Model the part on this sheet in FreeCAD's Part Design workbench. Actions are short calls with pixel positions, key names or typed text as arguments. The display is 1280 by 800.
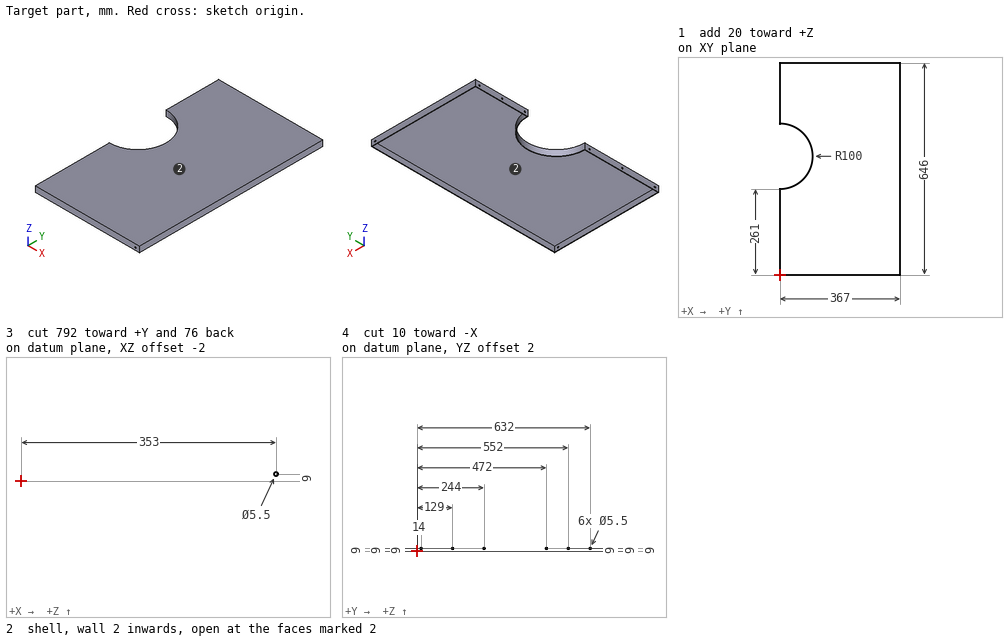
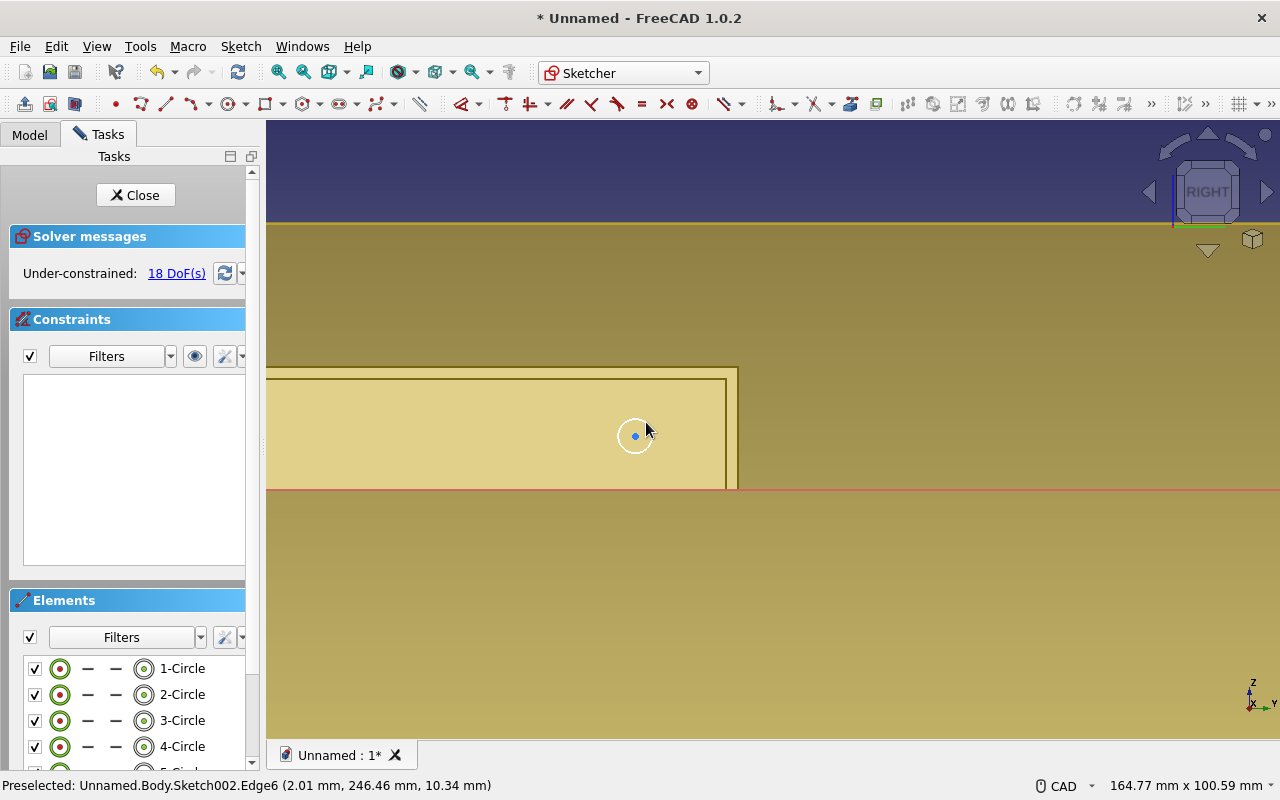
scroll(645, 426, down, 10)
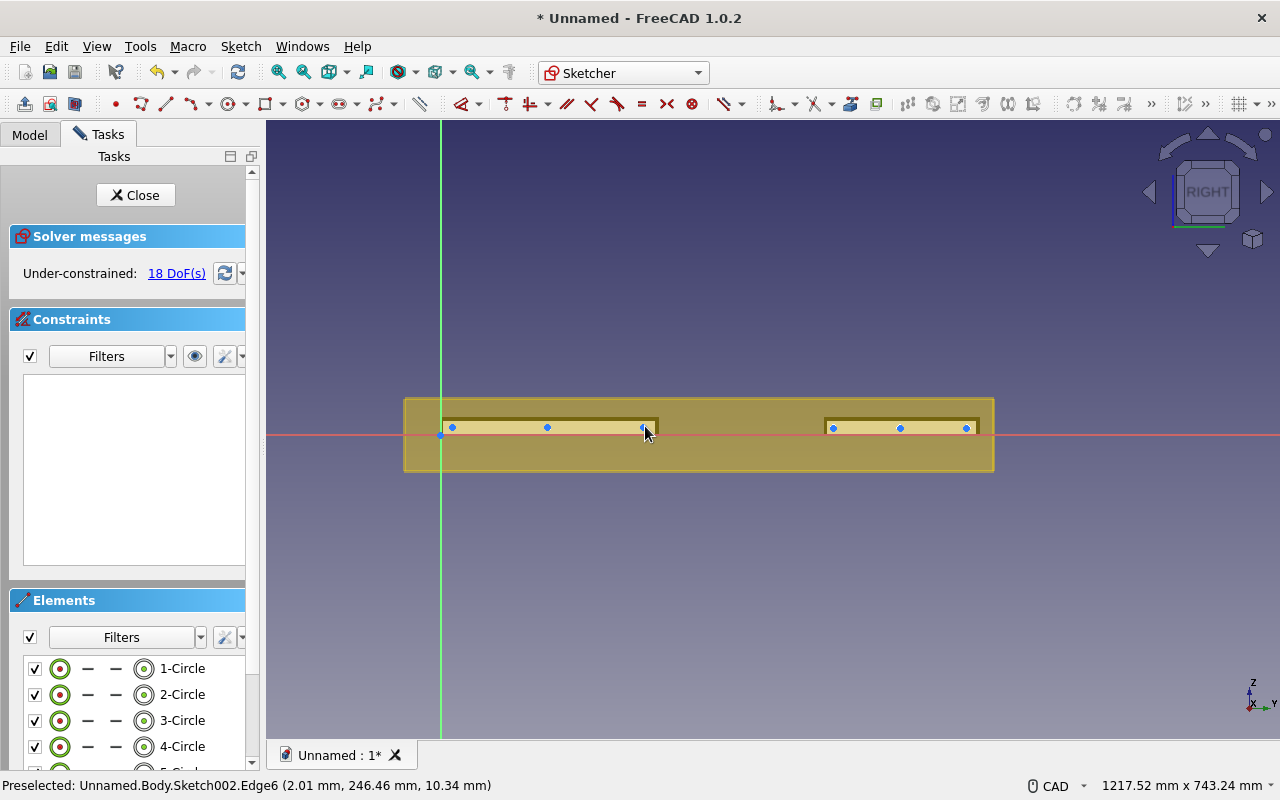
scroll(969, 426, up, 9)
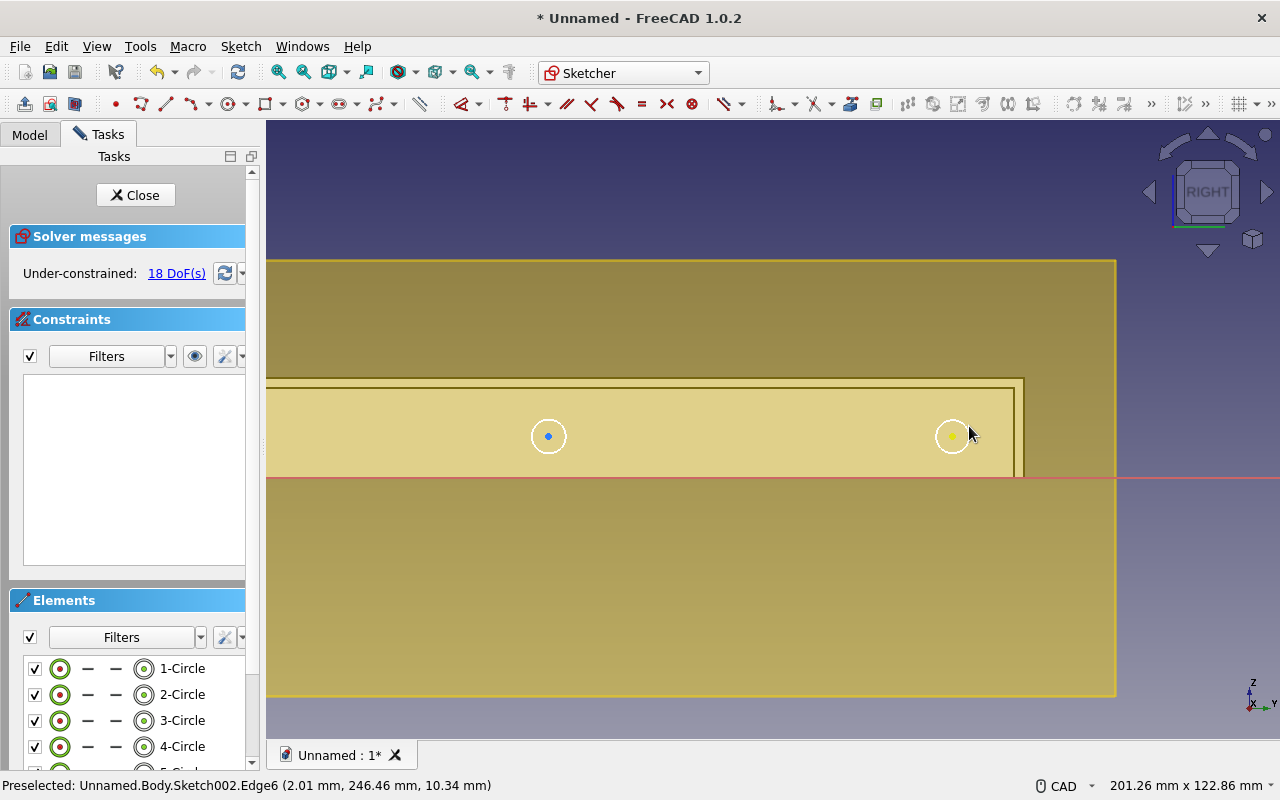
click(964, 425)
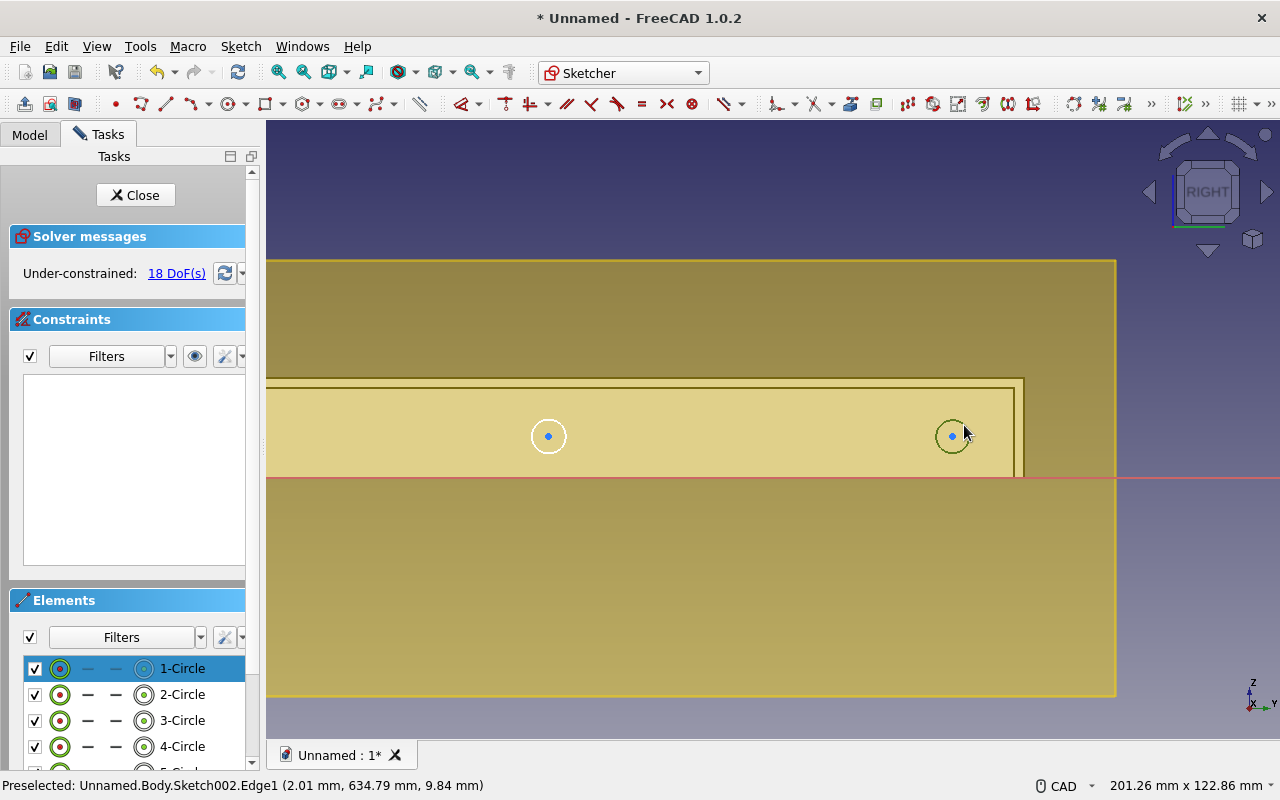
click(561, 424)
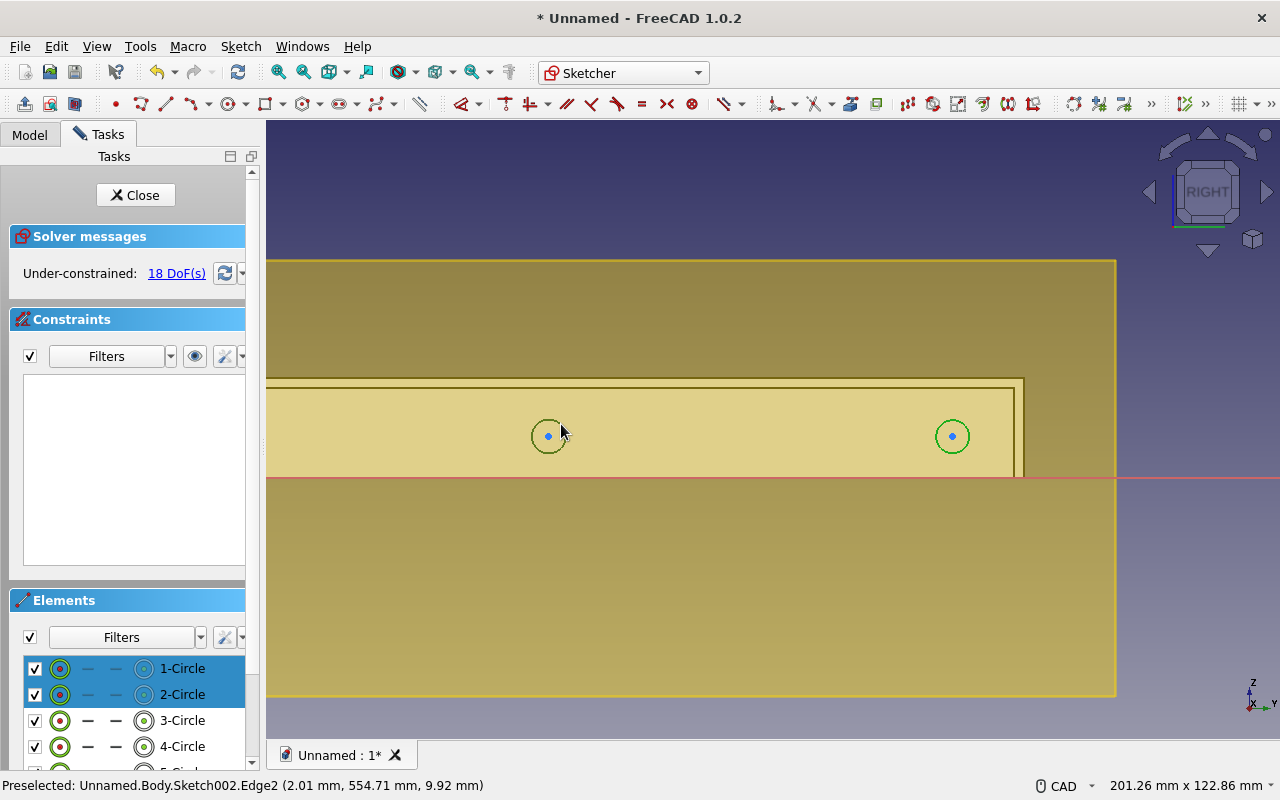
scroll(969, 426, down, 9)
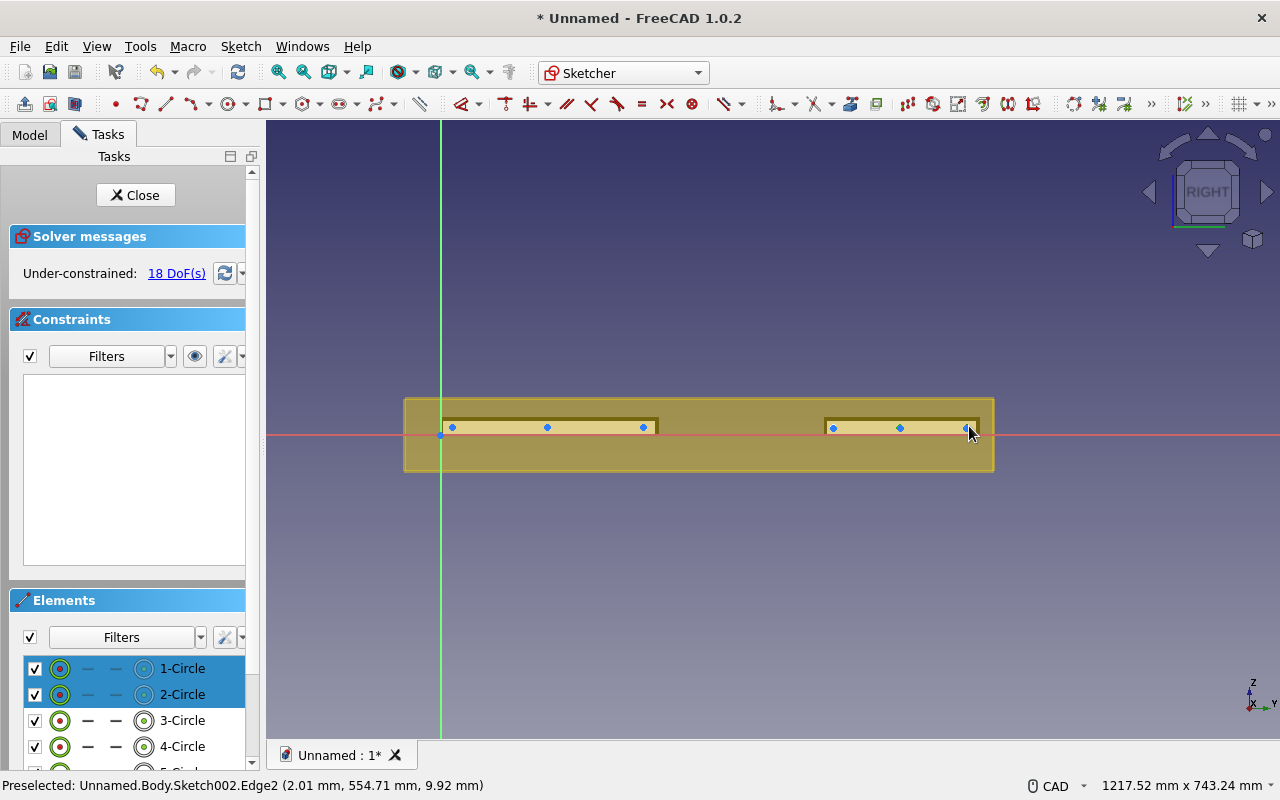
scroll(835, 426, up, 9)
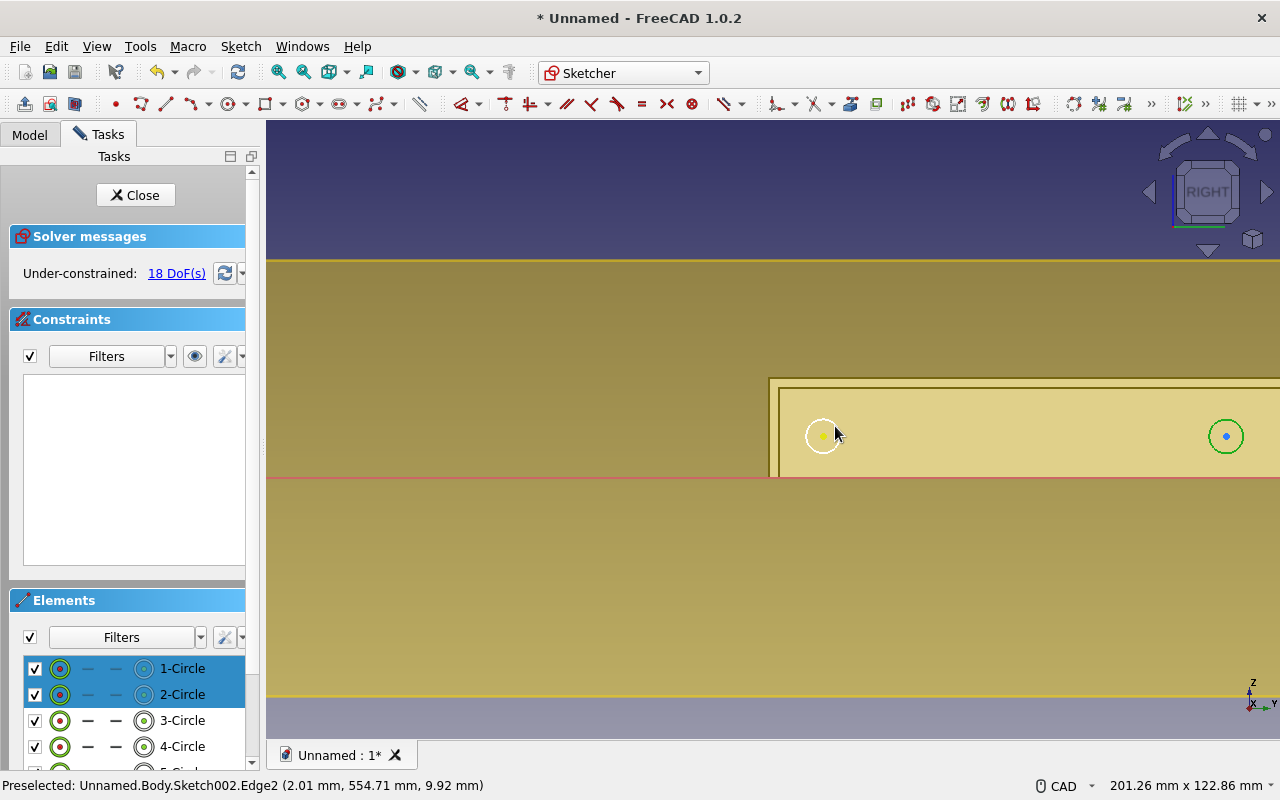
click(835, 424)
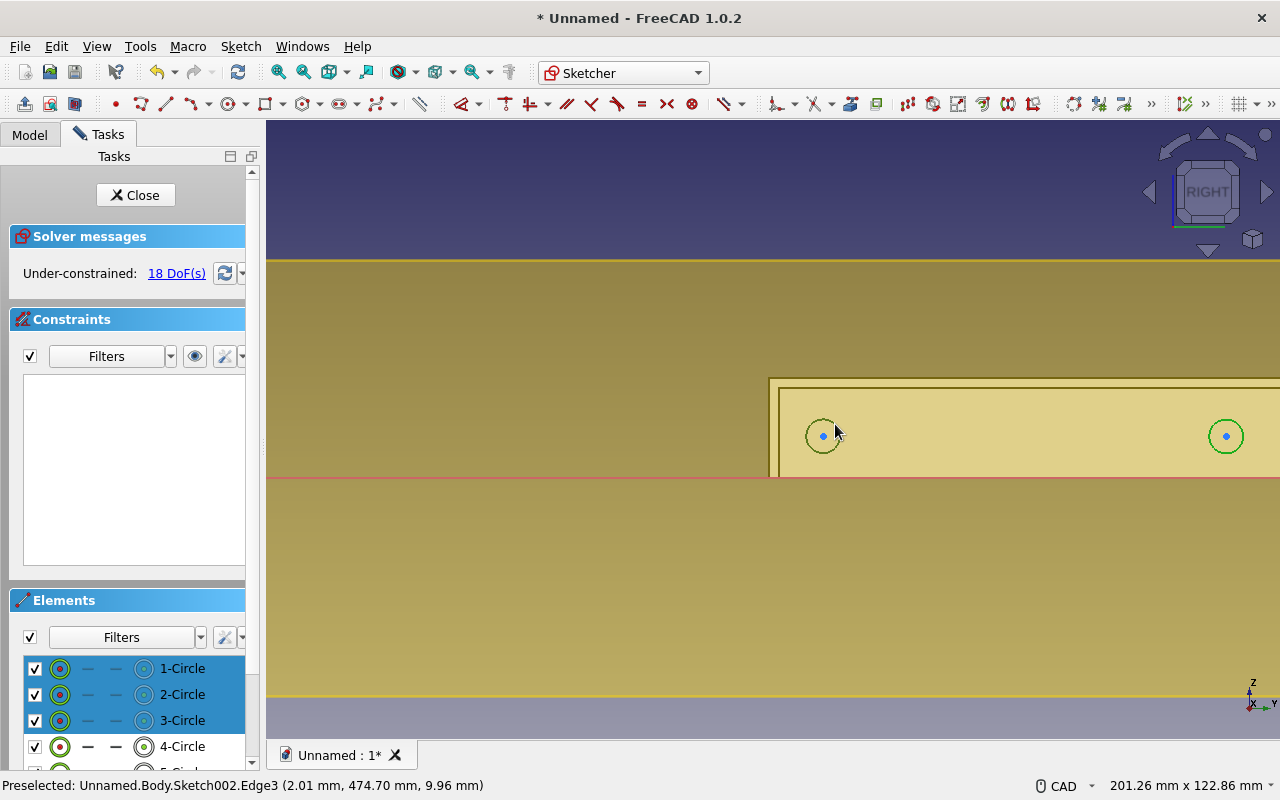
scroll(835, 426, down, 9)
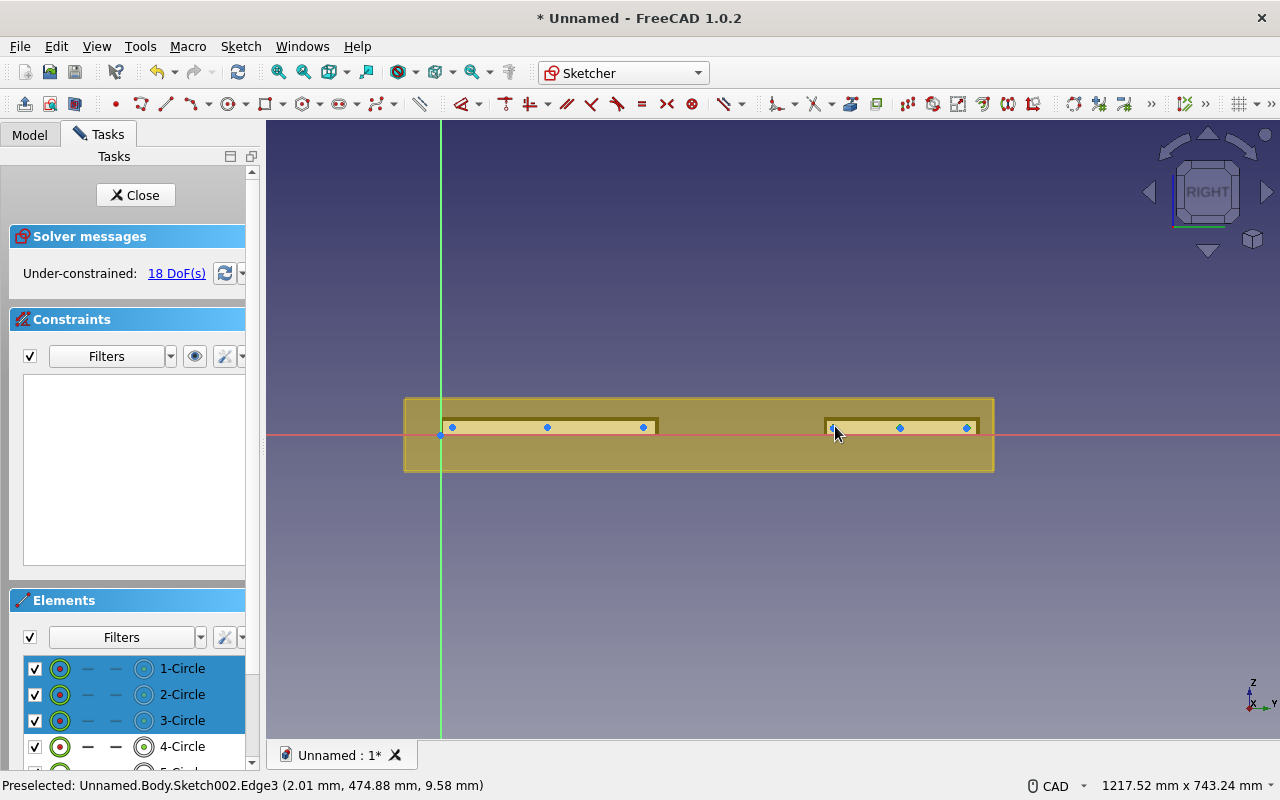
scroll(454, 426, up, 9)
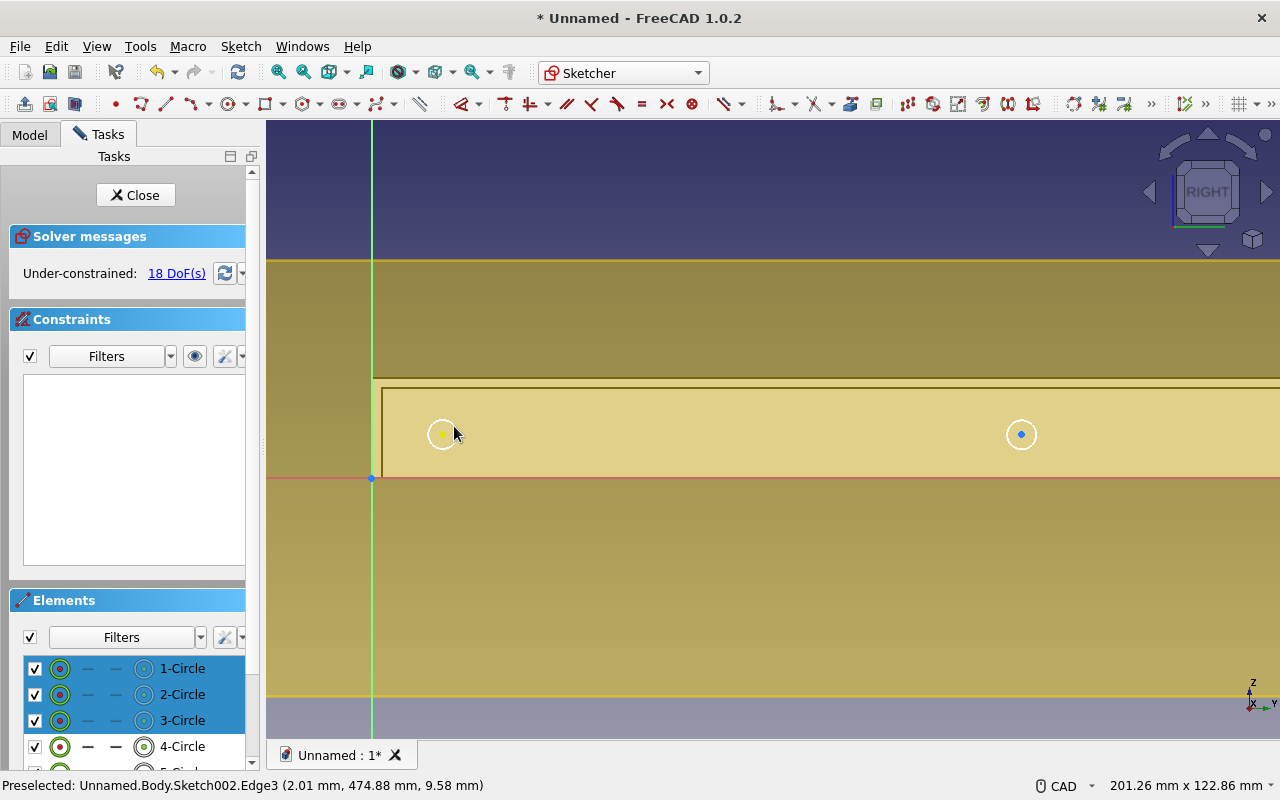
click(453, 424)